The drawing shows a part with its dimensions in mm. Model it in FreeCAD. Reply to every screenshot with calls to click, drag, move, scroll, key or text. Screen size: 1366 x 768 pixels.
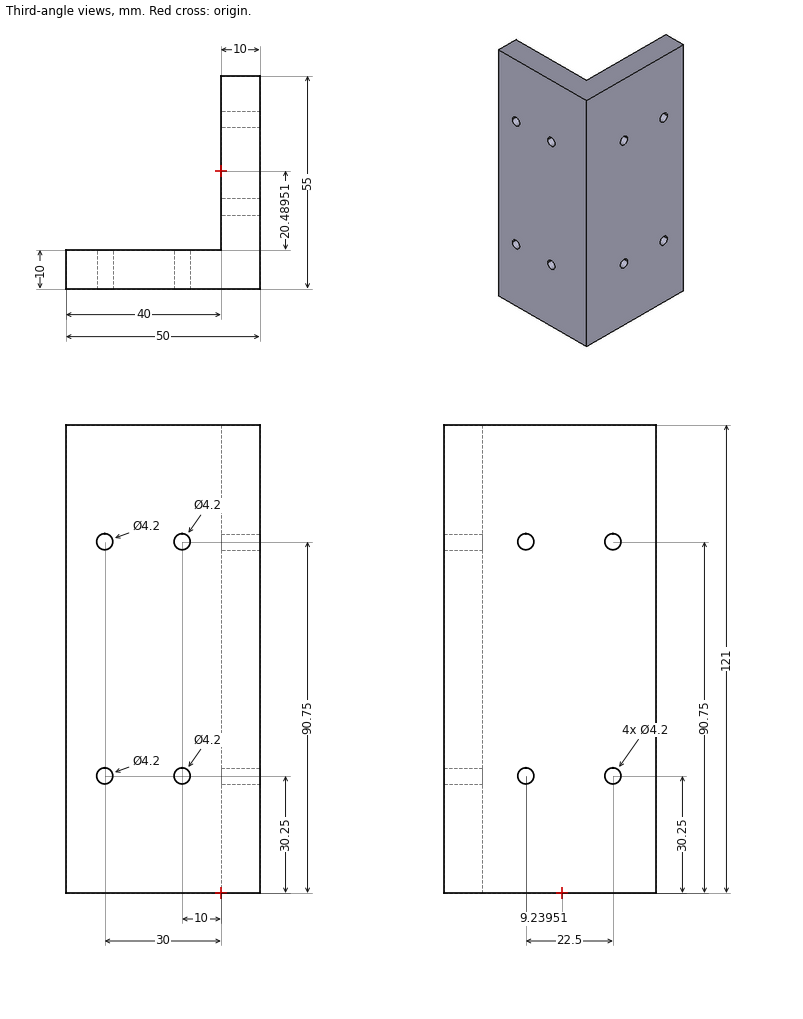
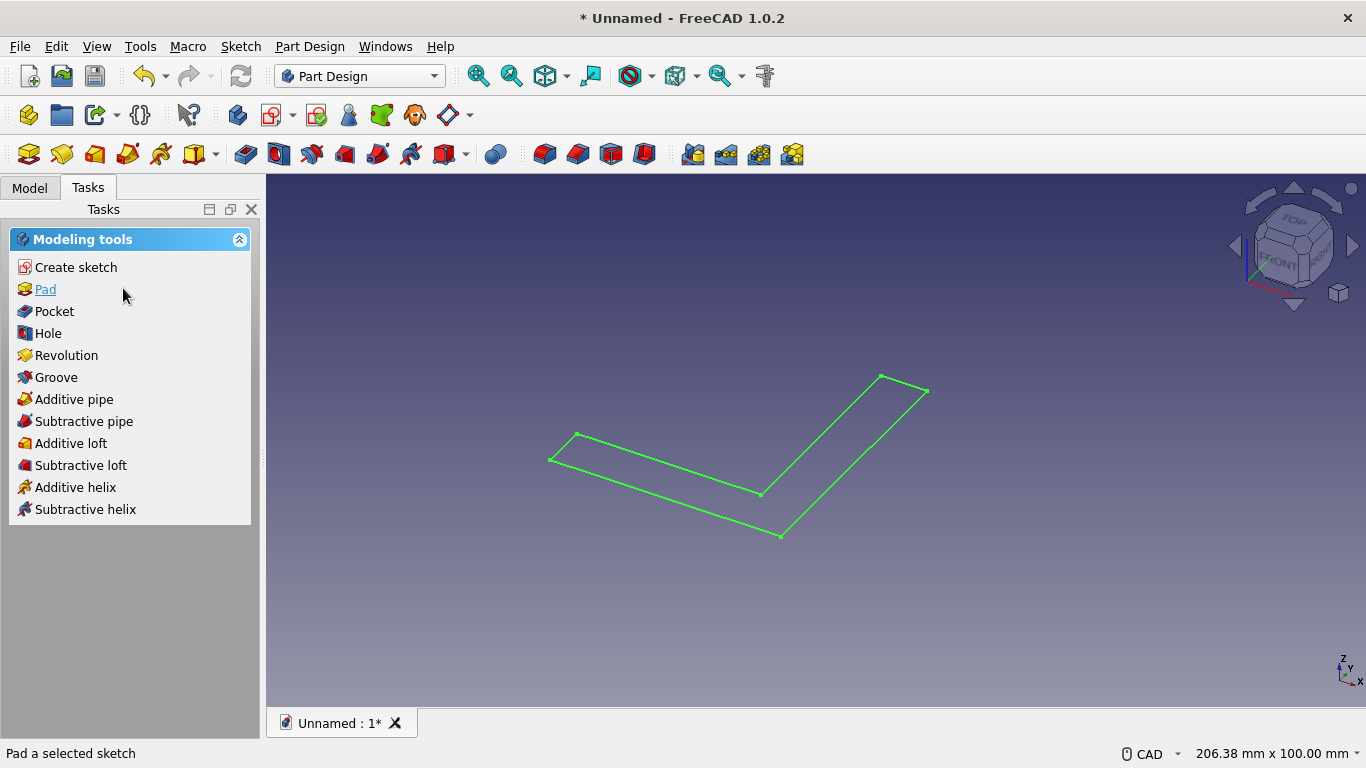
click(29, 154)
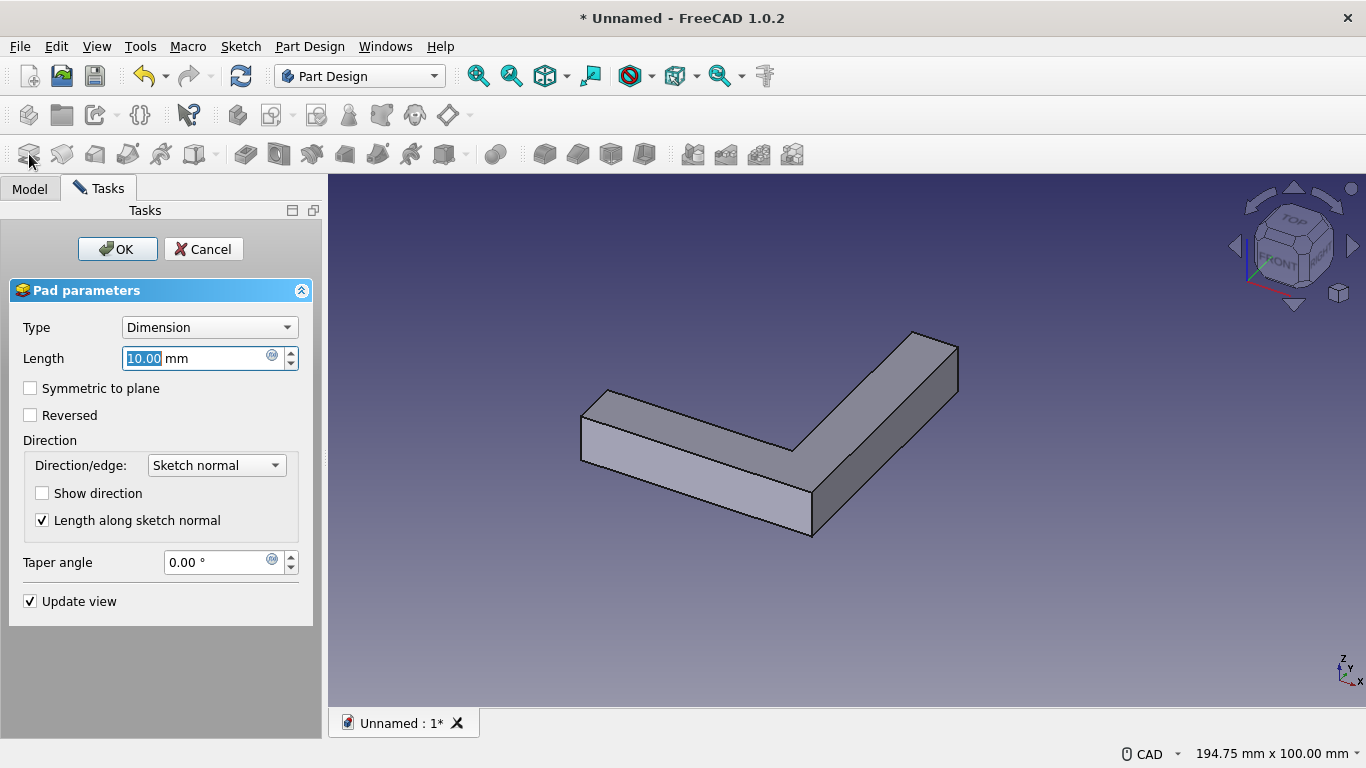
text(121)
key(Tab)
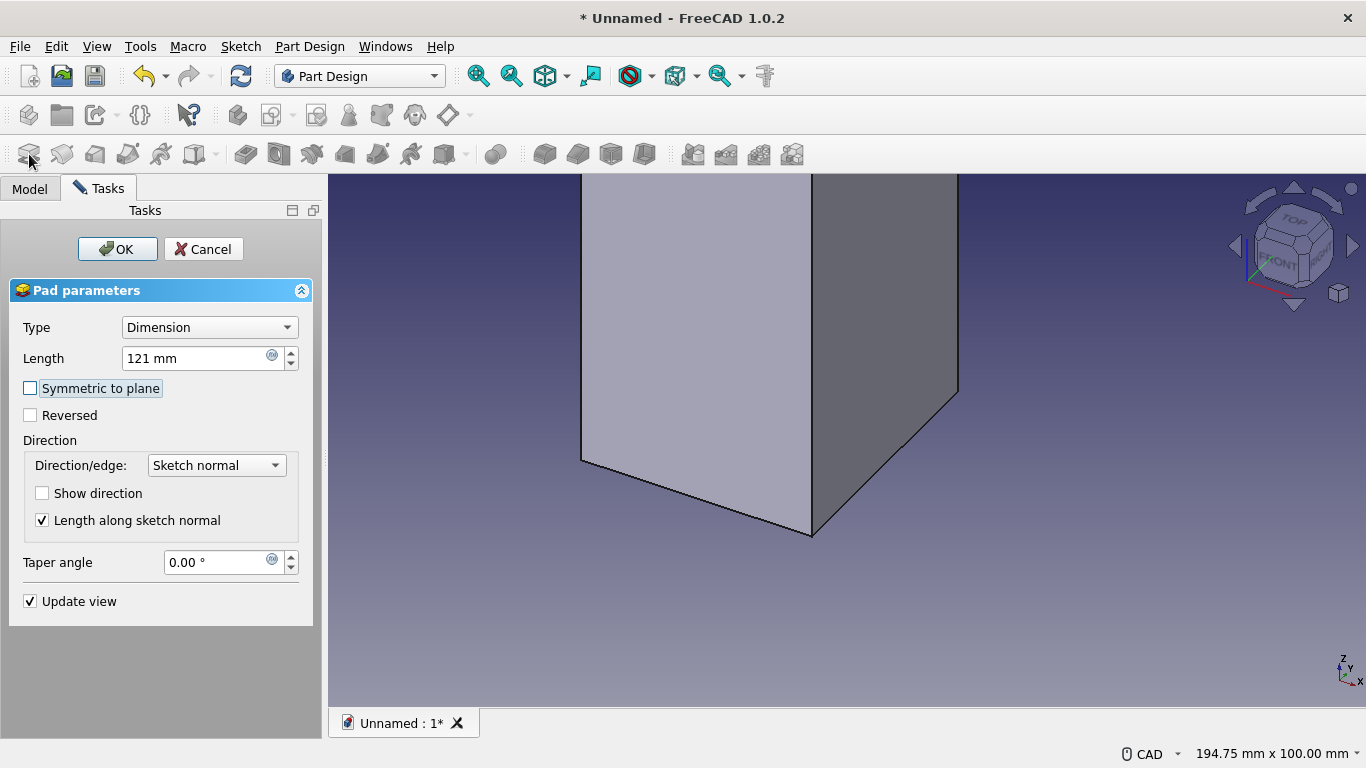
click(118, 249)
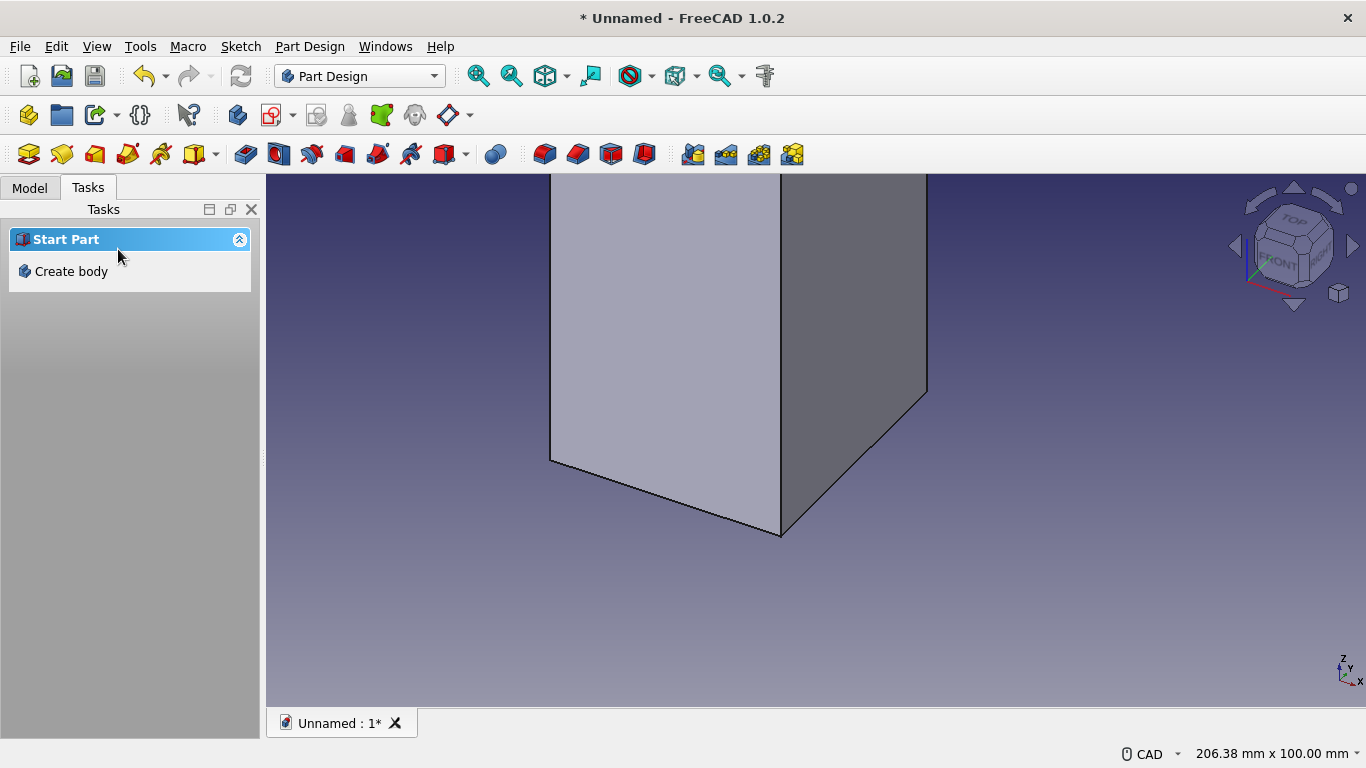
key(v)
key(f)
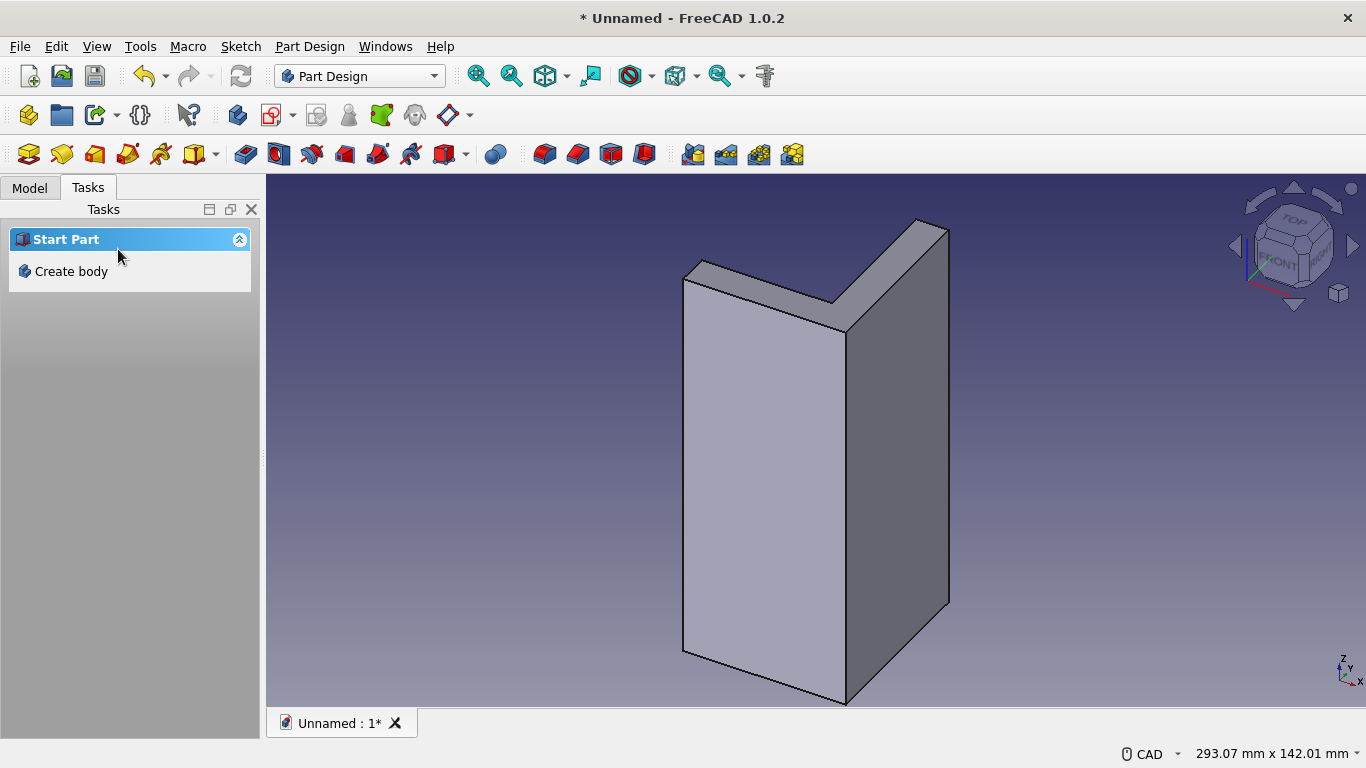
key(4)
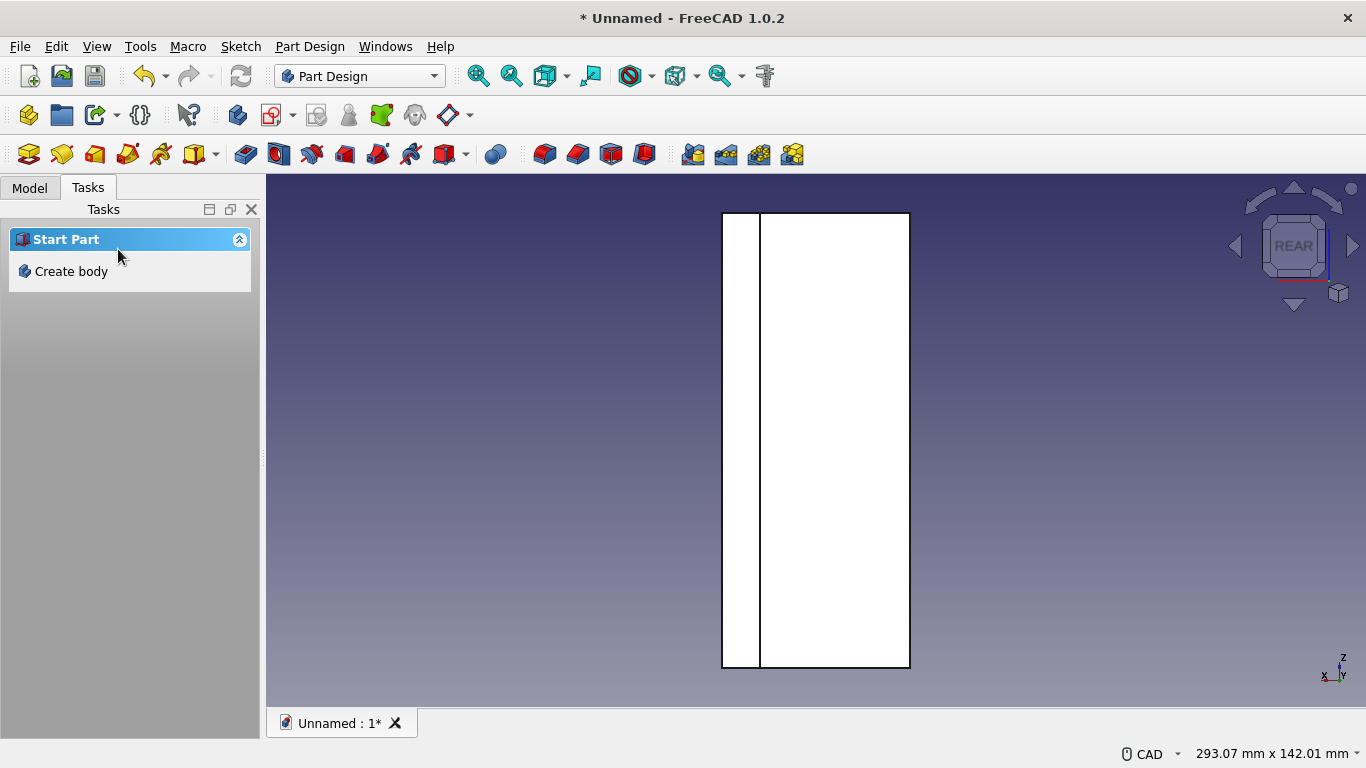
click(835, 310)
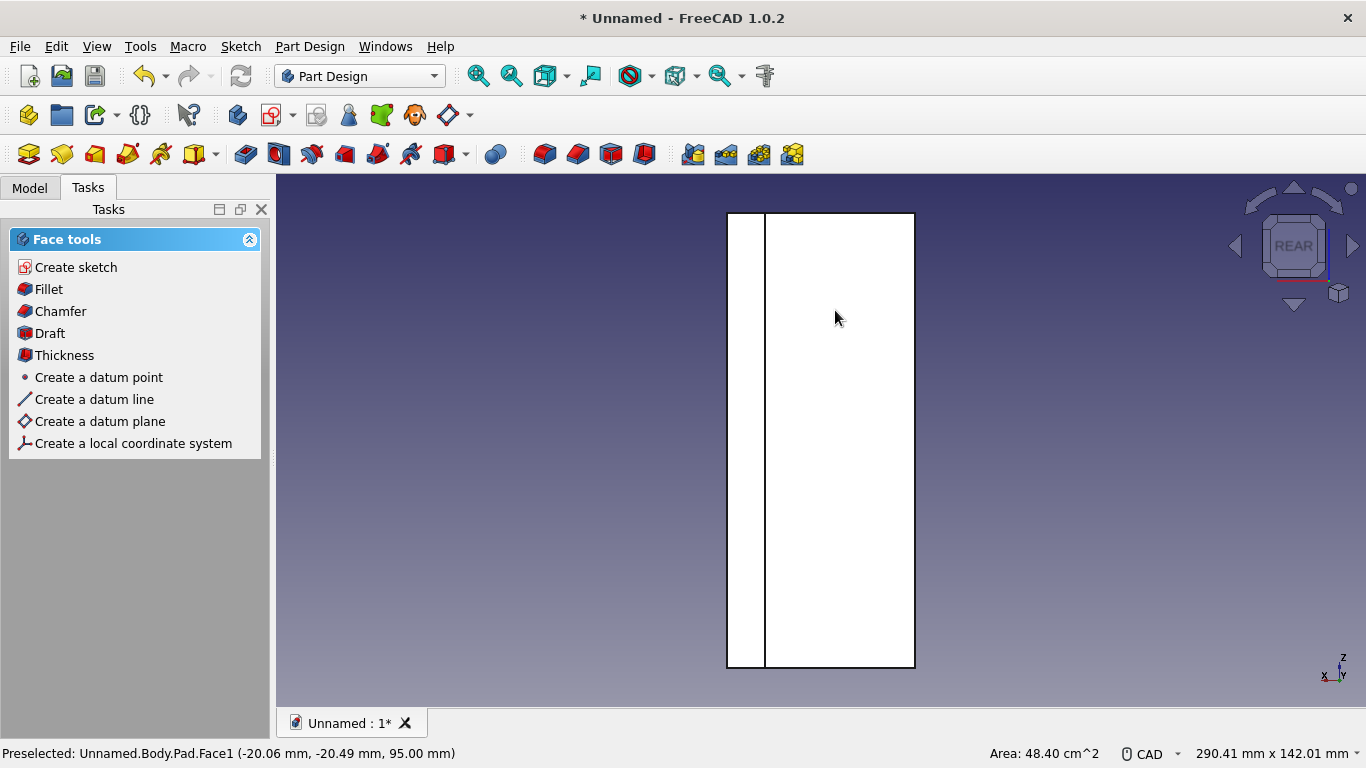
click(270, 116)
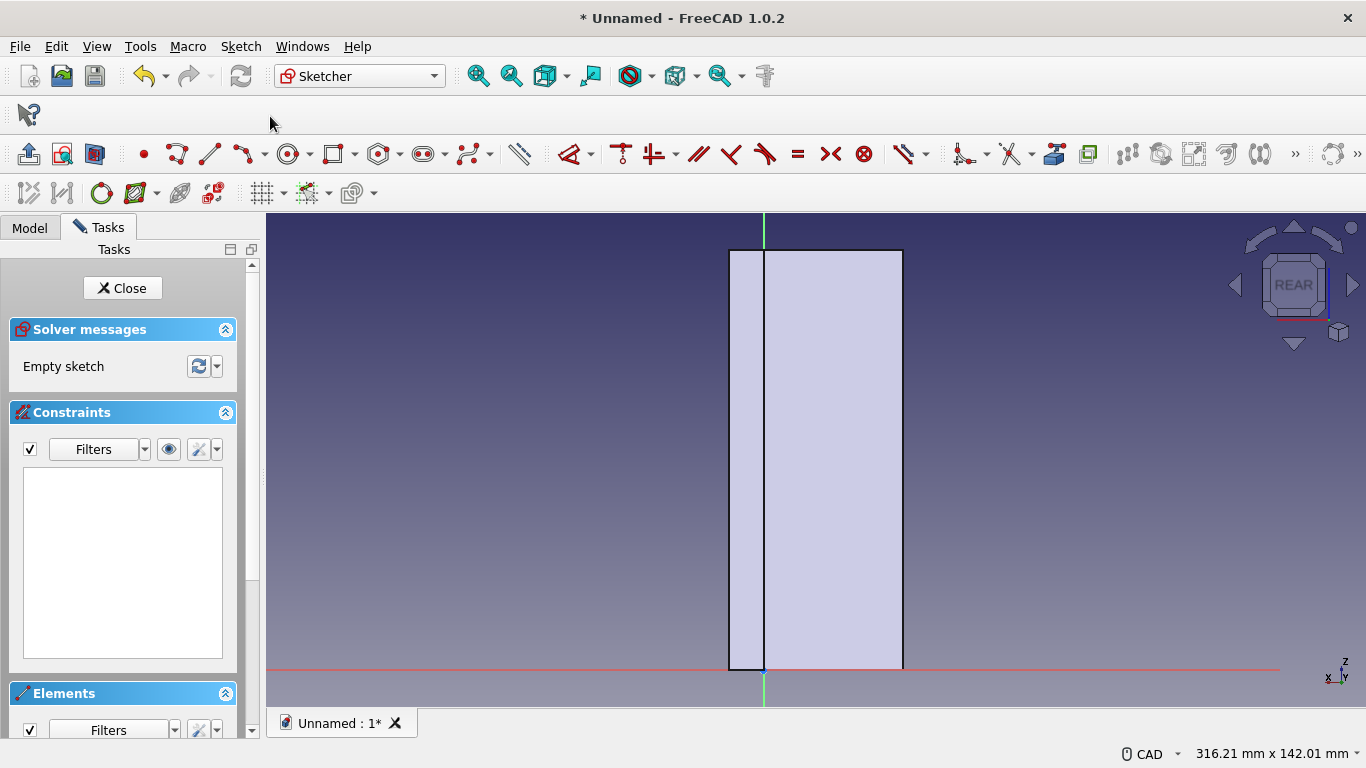
scroll(801, 349, up, 15)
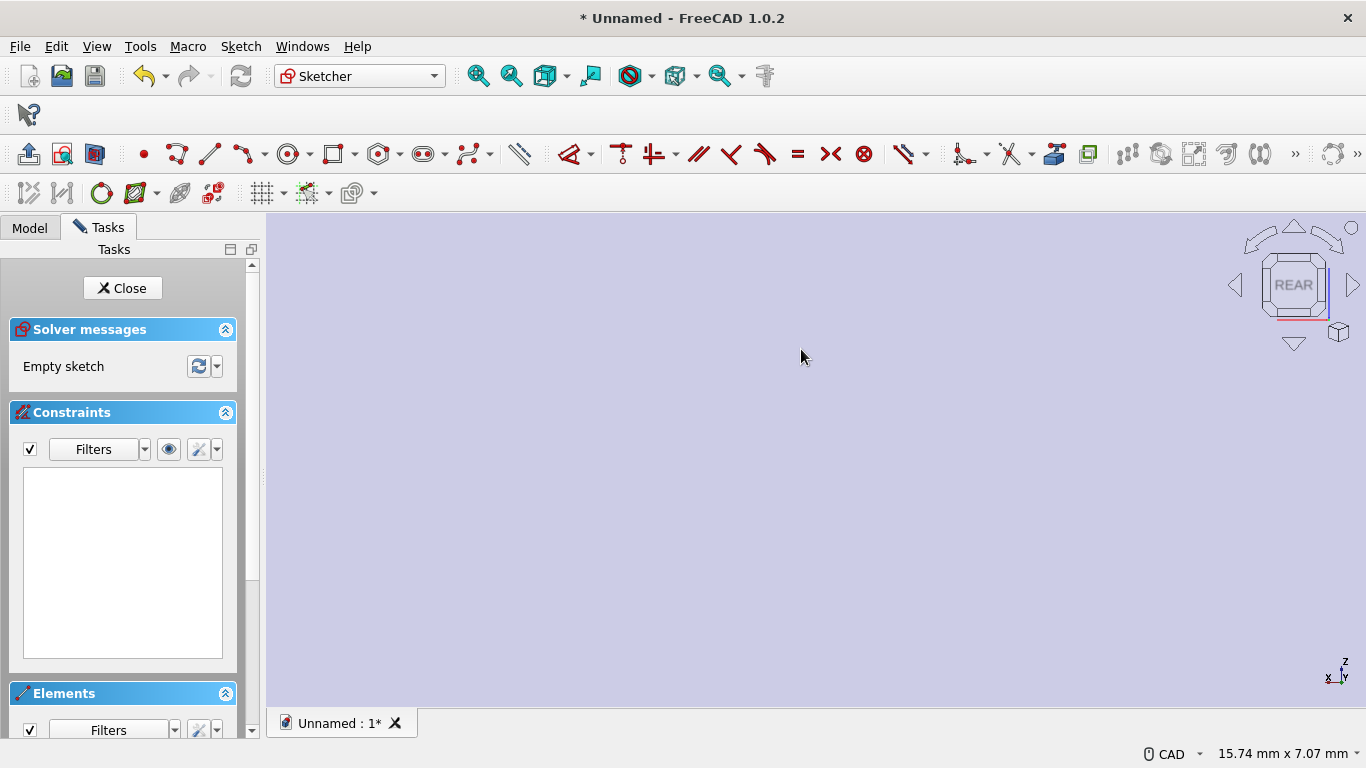
key(g)
key(c)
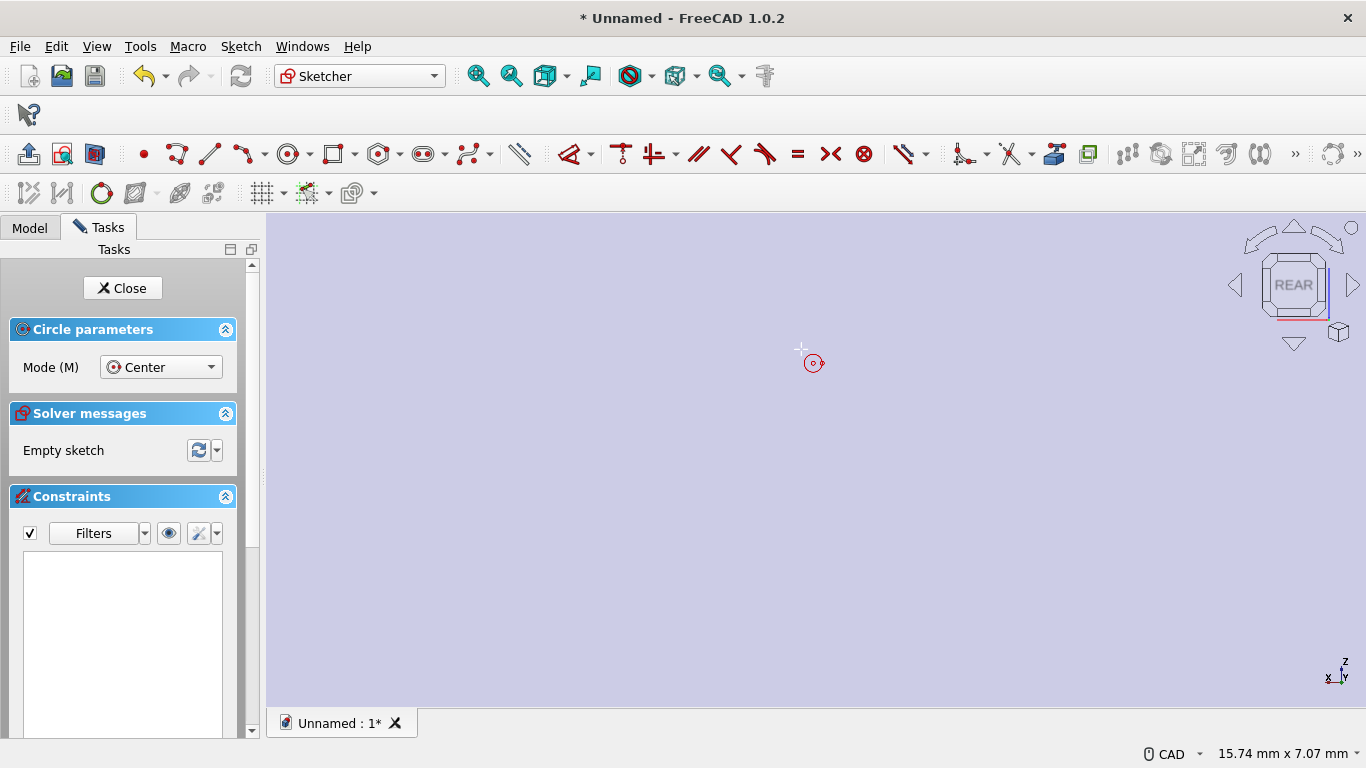
click(744, 460)
move(847, 356)